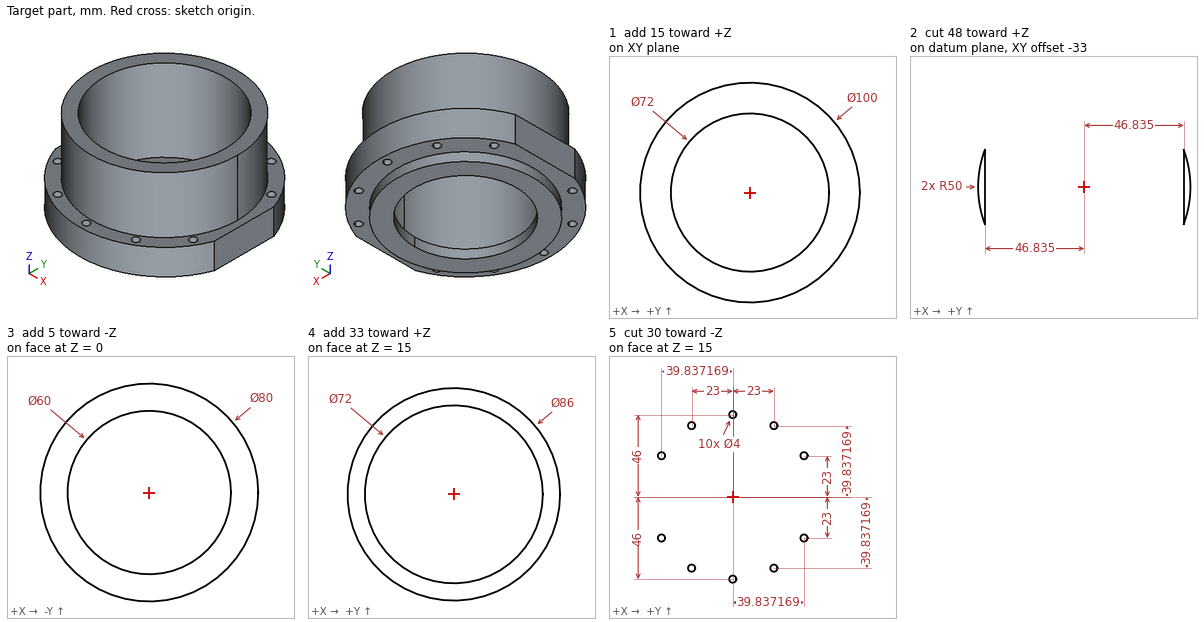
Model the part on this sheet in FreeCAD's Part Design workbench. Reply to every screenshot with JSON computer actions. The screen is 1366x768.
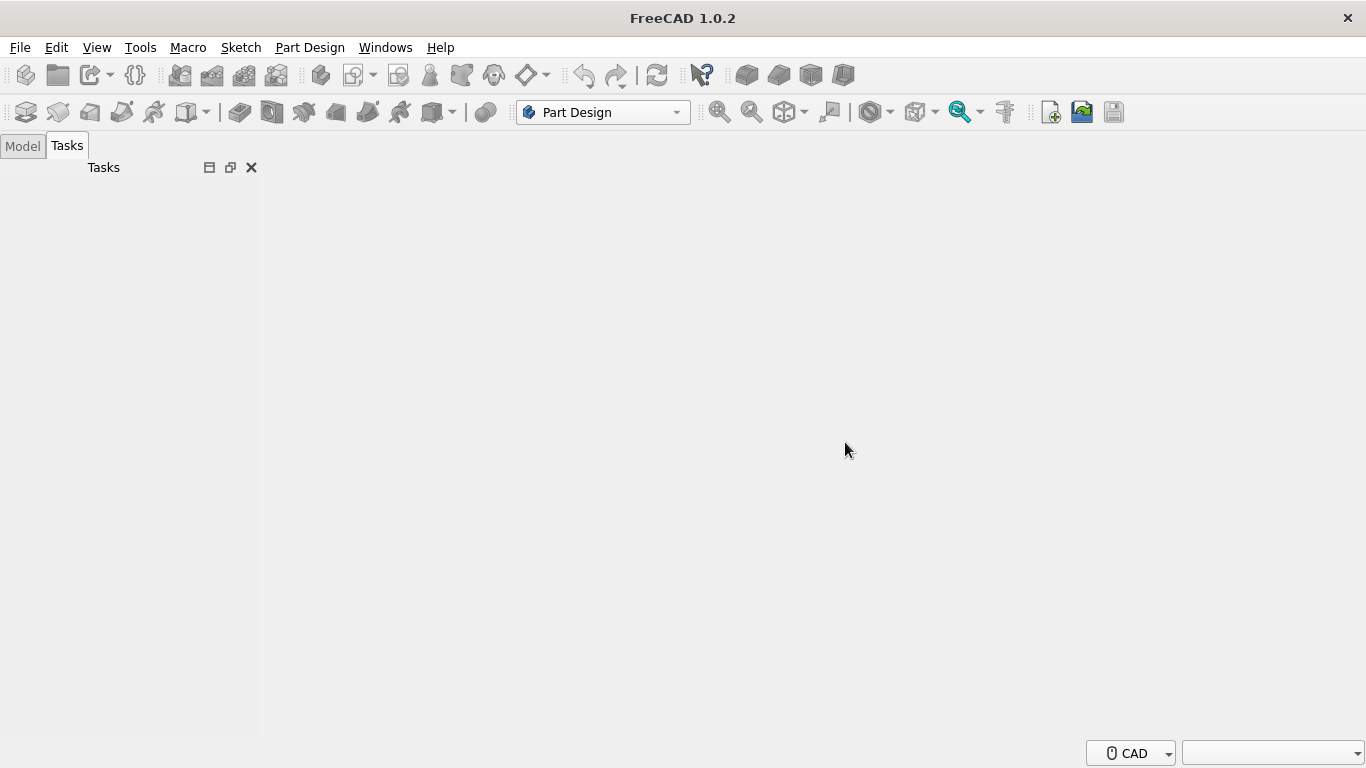
{"action": "left_click", "coordinate": [1050, 112]}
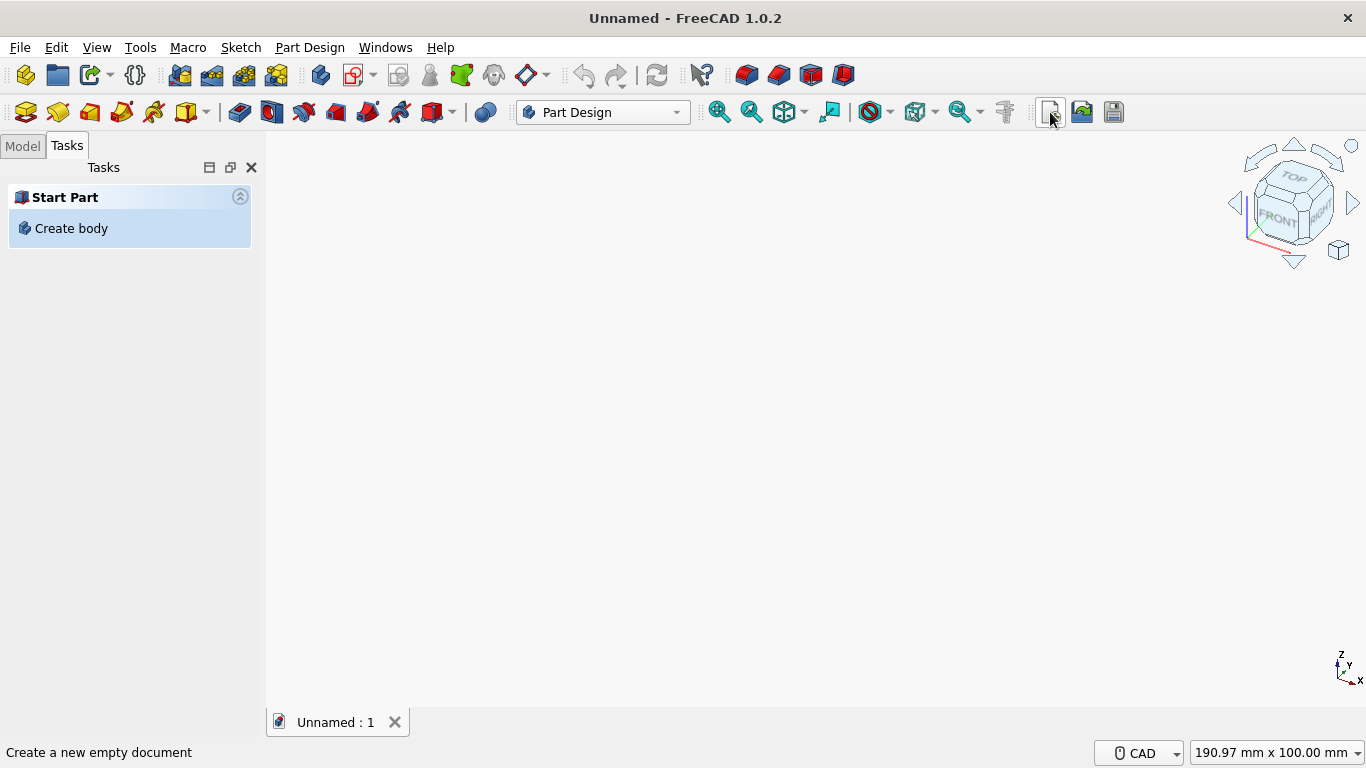
{"action": "left_click", "coordinate": [354, 76]}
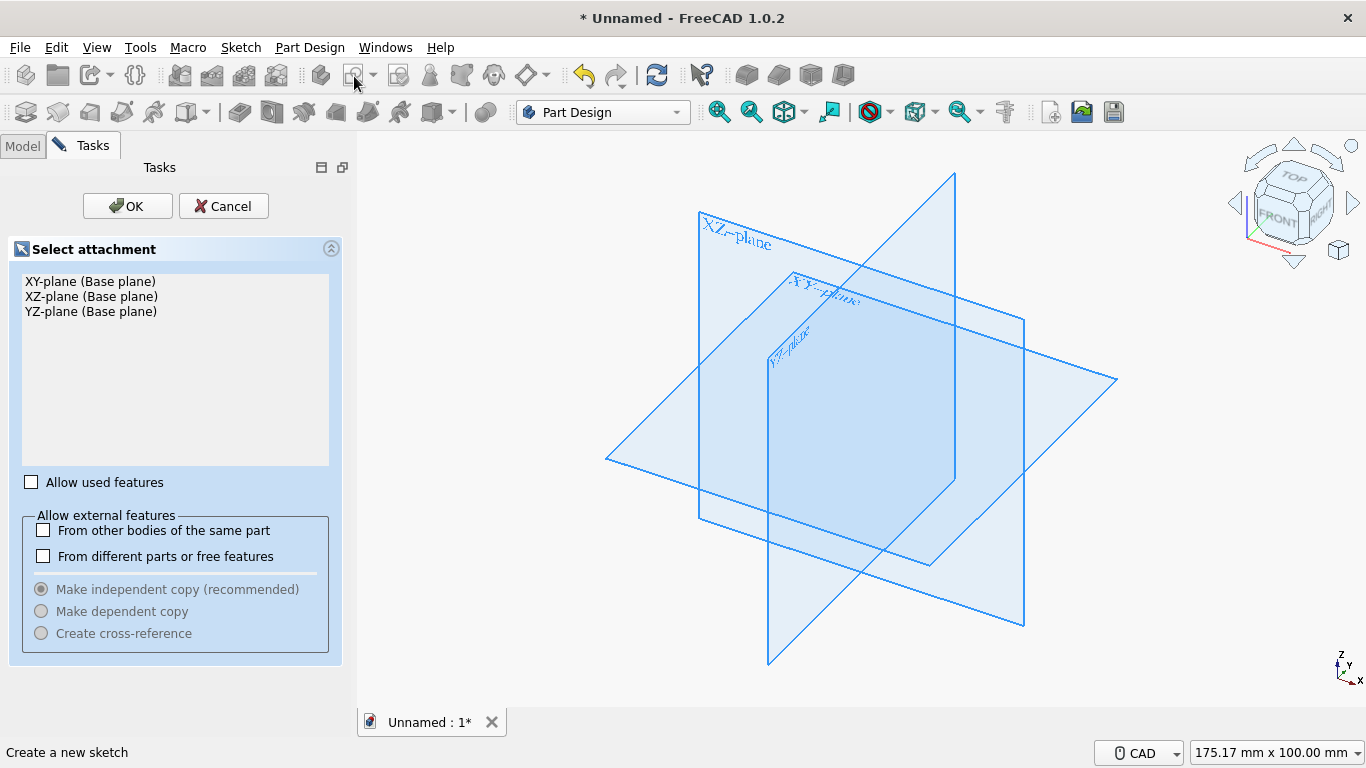
{"action": "left_click", "coordinate": [82, 282]}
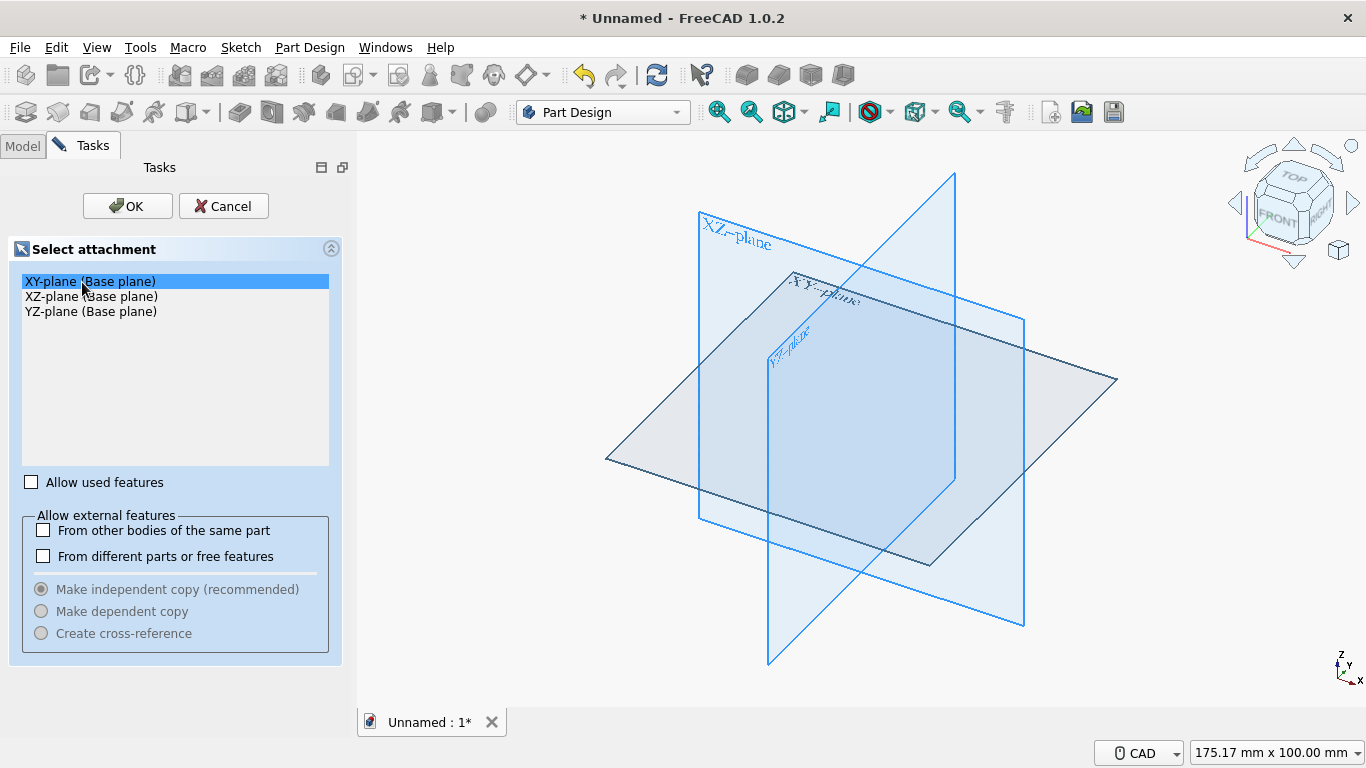
{"action": "left_click", "coordinate": [128, 206]}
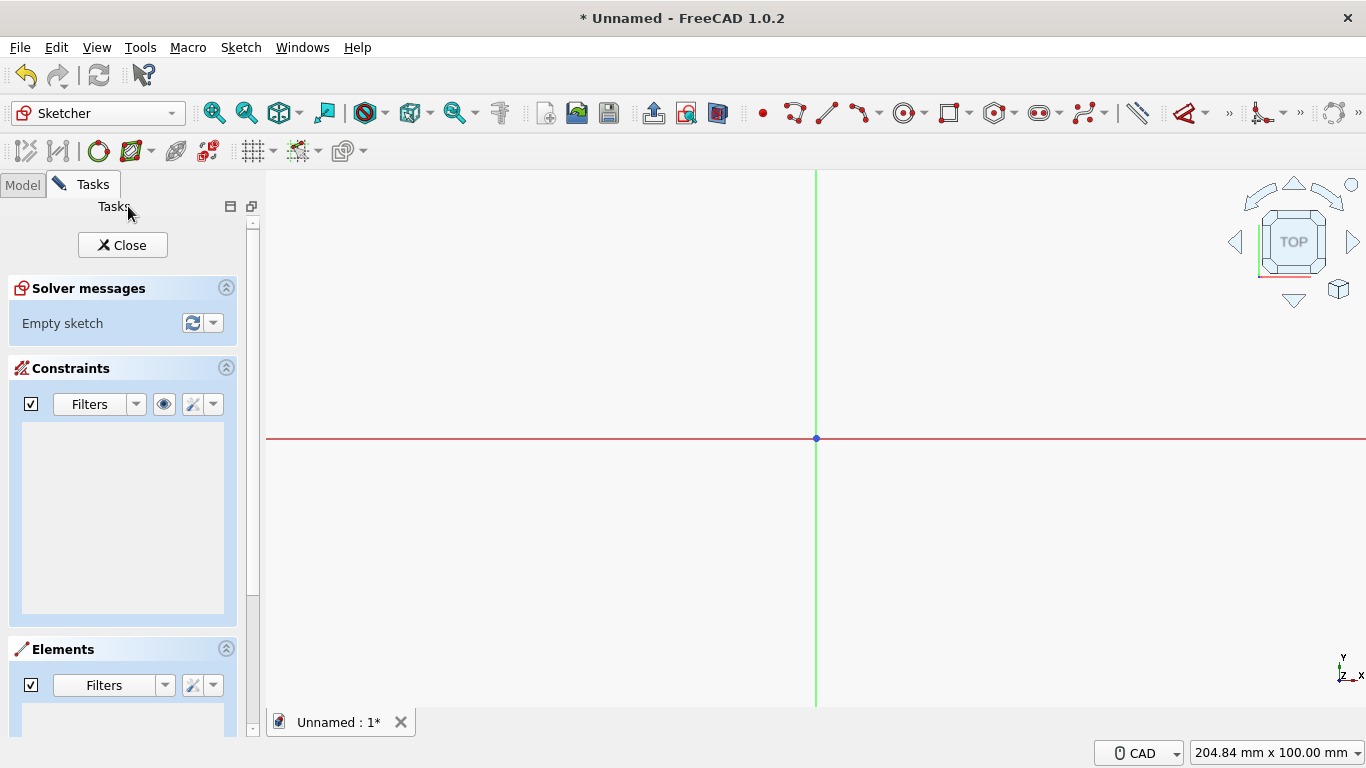
{"action": "scroll", "coordinate": [608, 438], "scroll_direction": "down", "scroll_amount": 2}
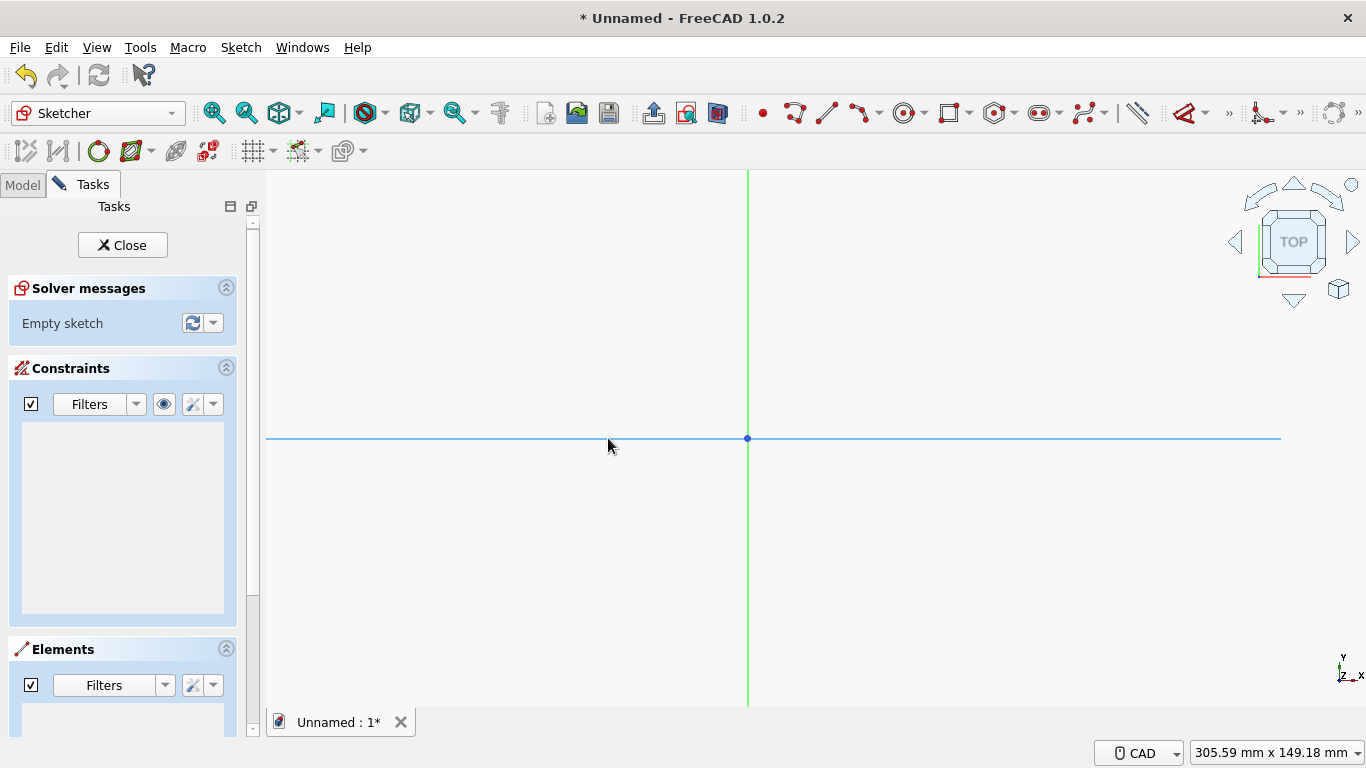
{"action": "left_click", "coordinate": [904, 114]}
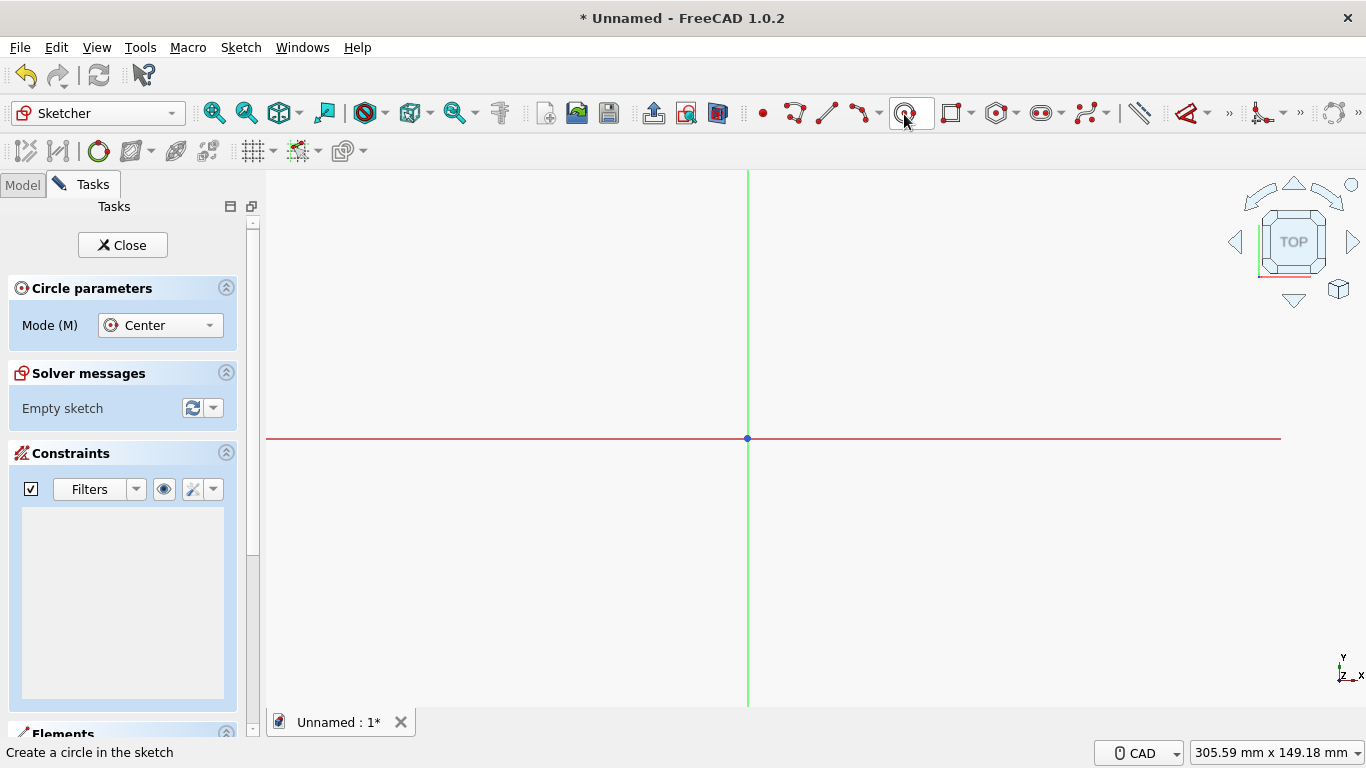
{"action": "left_click", "coordinate": [748, 438]}
{"action": "mouse_move", "coordinate": [875, 311]}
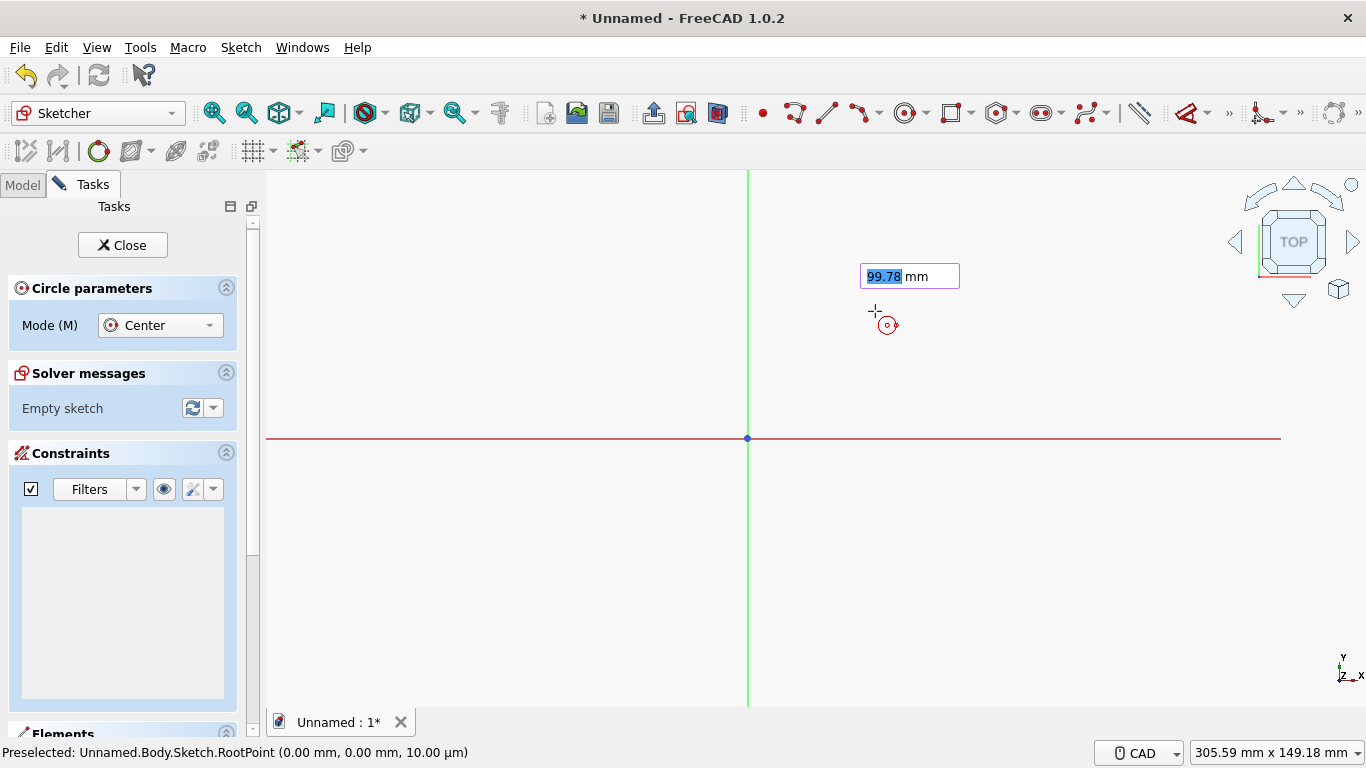
{"action": "type", "text": "100"}
{"action": "key", "text": "Return"}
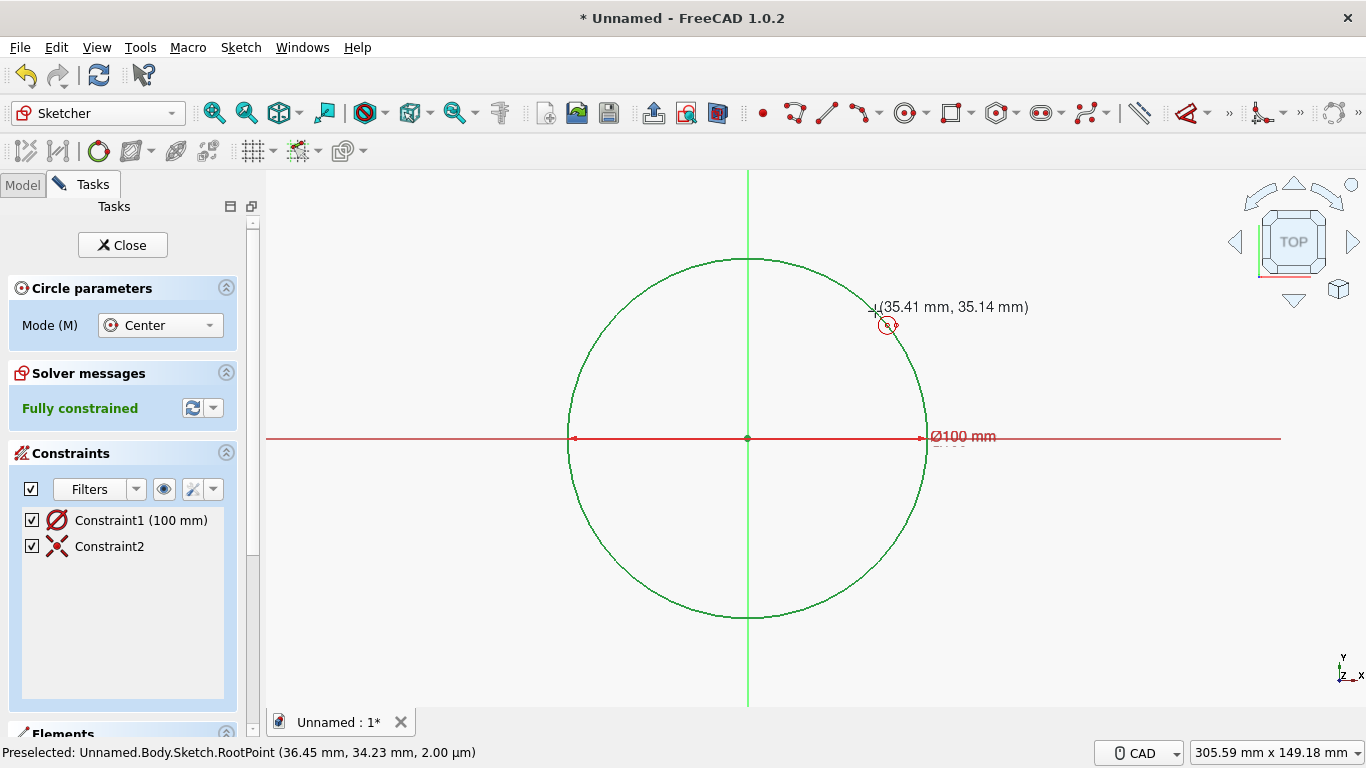
{"action": "left_click", "coordinate": [748, 438]}
{"action": "mouse_move", "coordinate": [839, 347]}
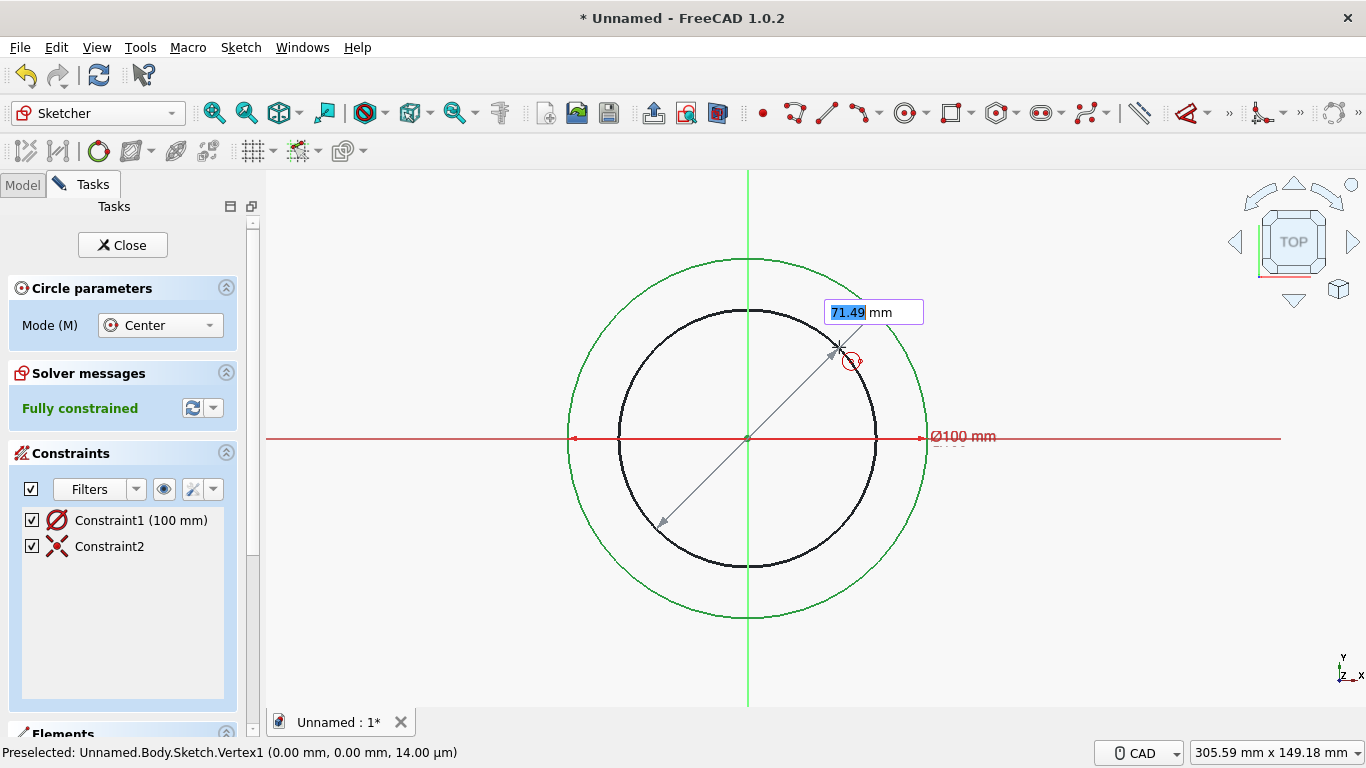
{"action": "type", "text": "72"}
{"action": "key", "text": "Return"}
{"action": "key", "text": "Escape"}